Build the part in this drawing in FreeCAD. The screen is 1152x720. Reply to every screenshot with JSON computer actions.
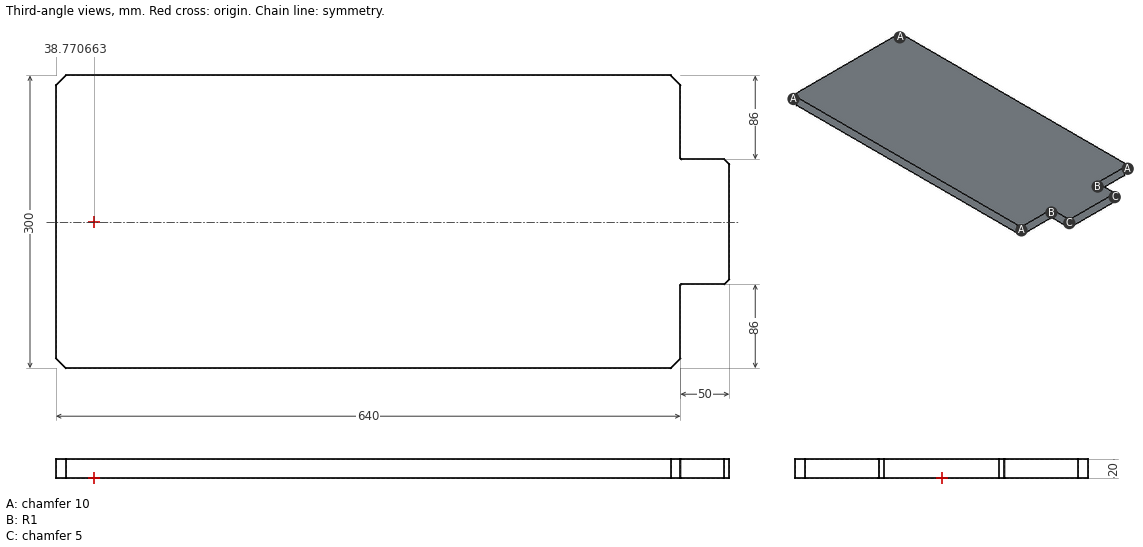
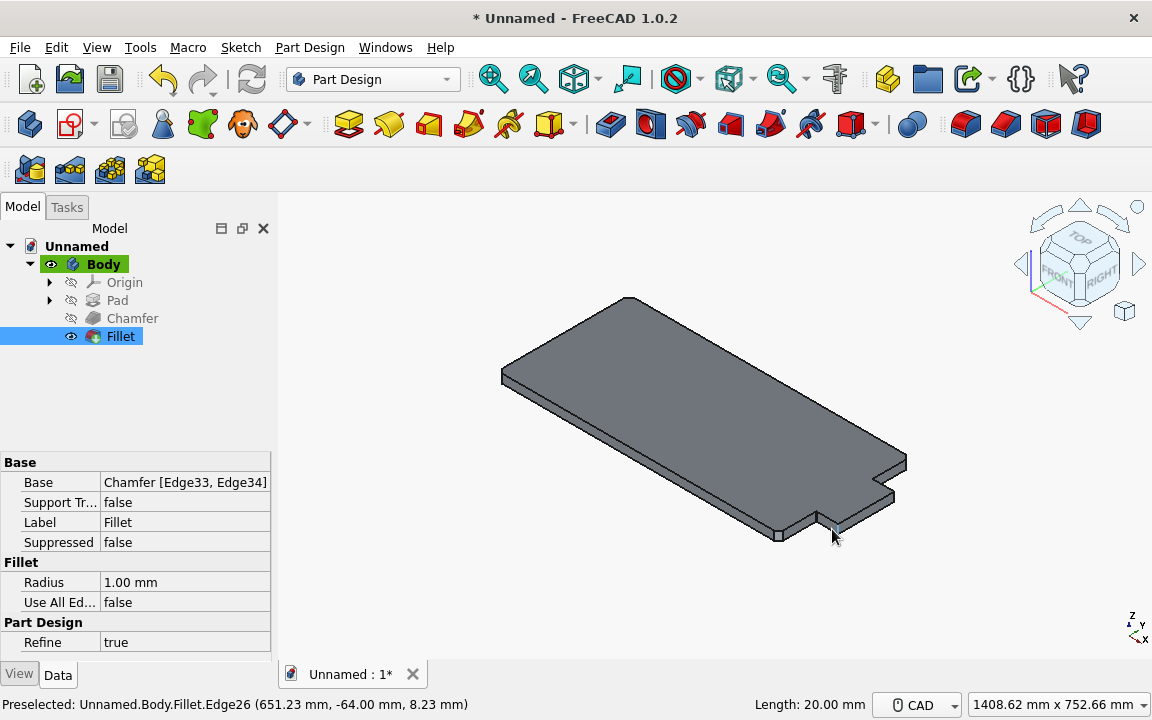
{"action": "scroll", "coordinate": [894, 496], "scroll_direction": "up", "scroll_amount": 6}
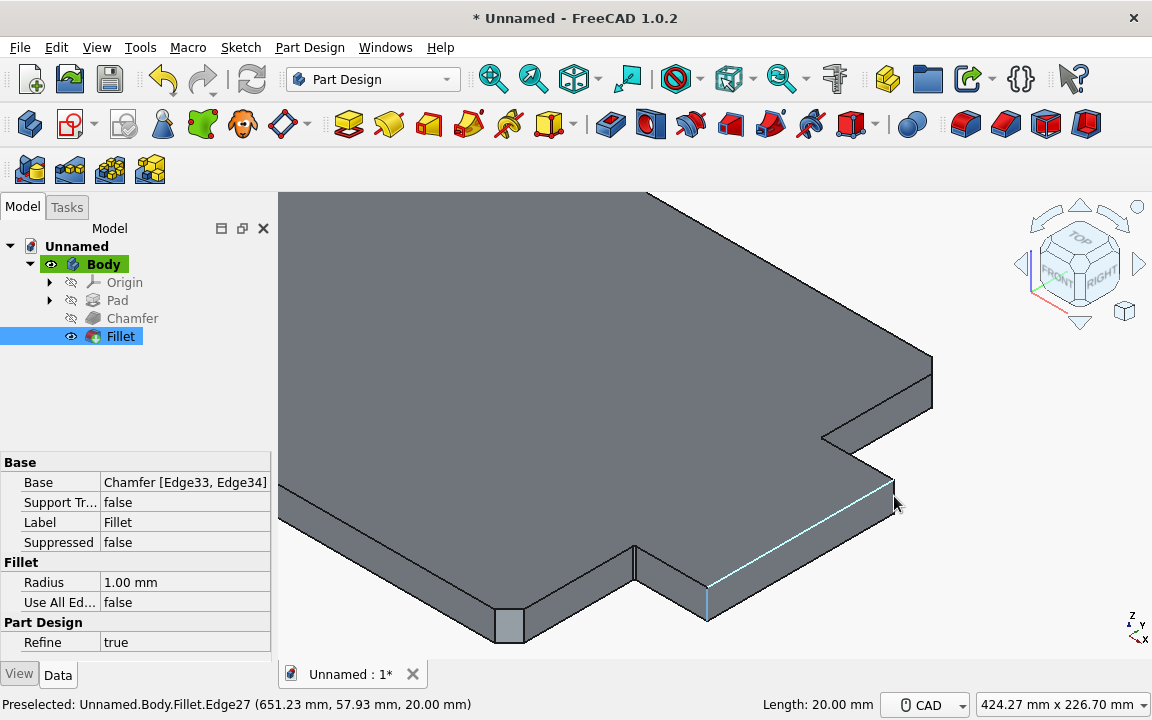
{"action": "left_click", "coordinate": [494, 80]}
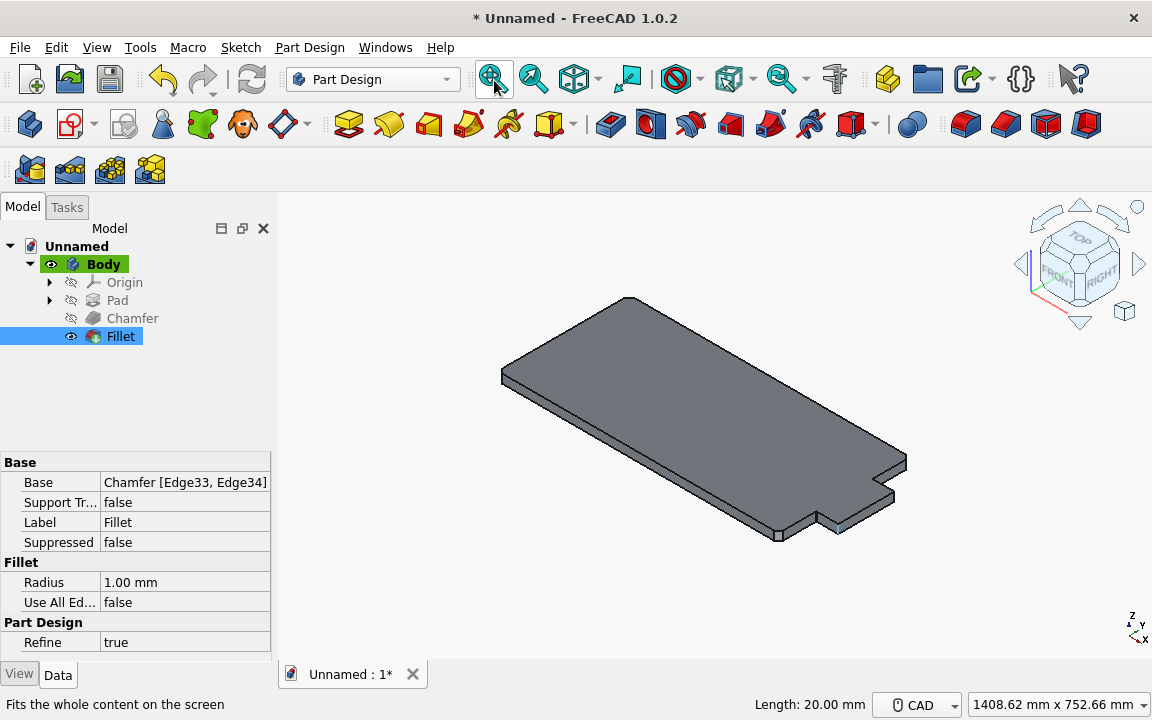
{"action": "key", "text": "2"}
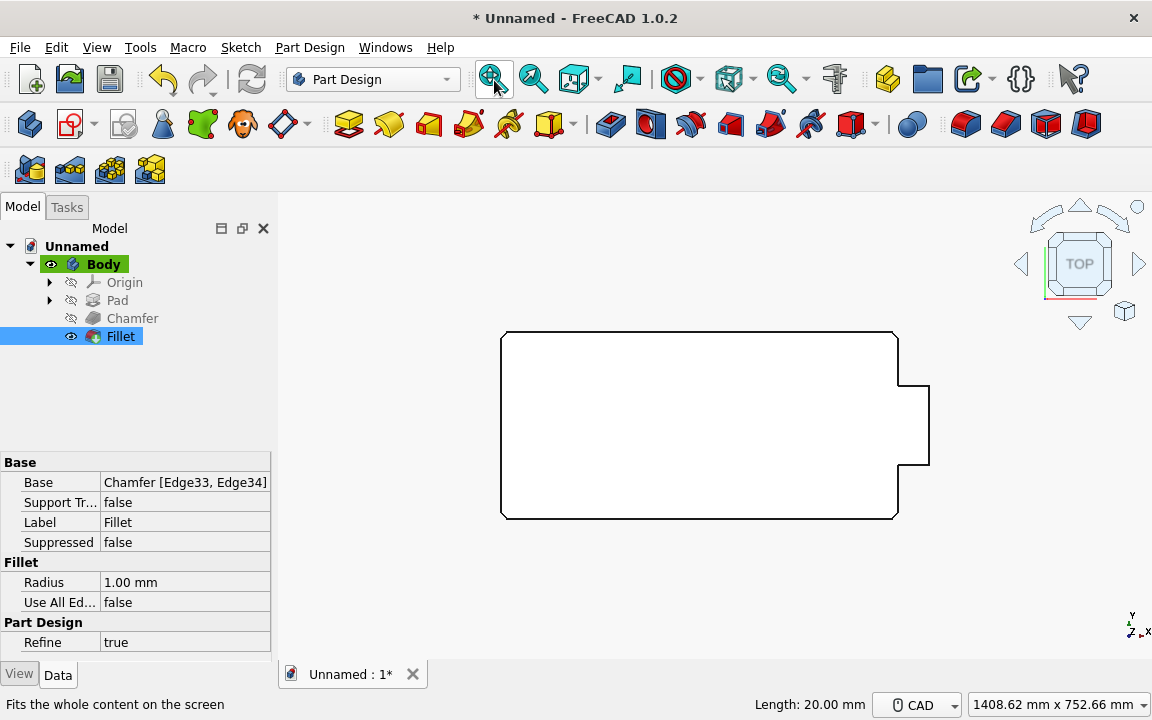
{"action": "scroll", "coordinate": [929, 385], "scroll_direction": "up", "scroll_amount": 6}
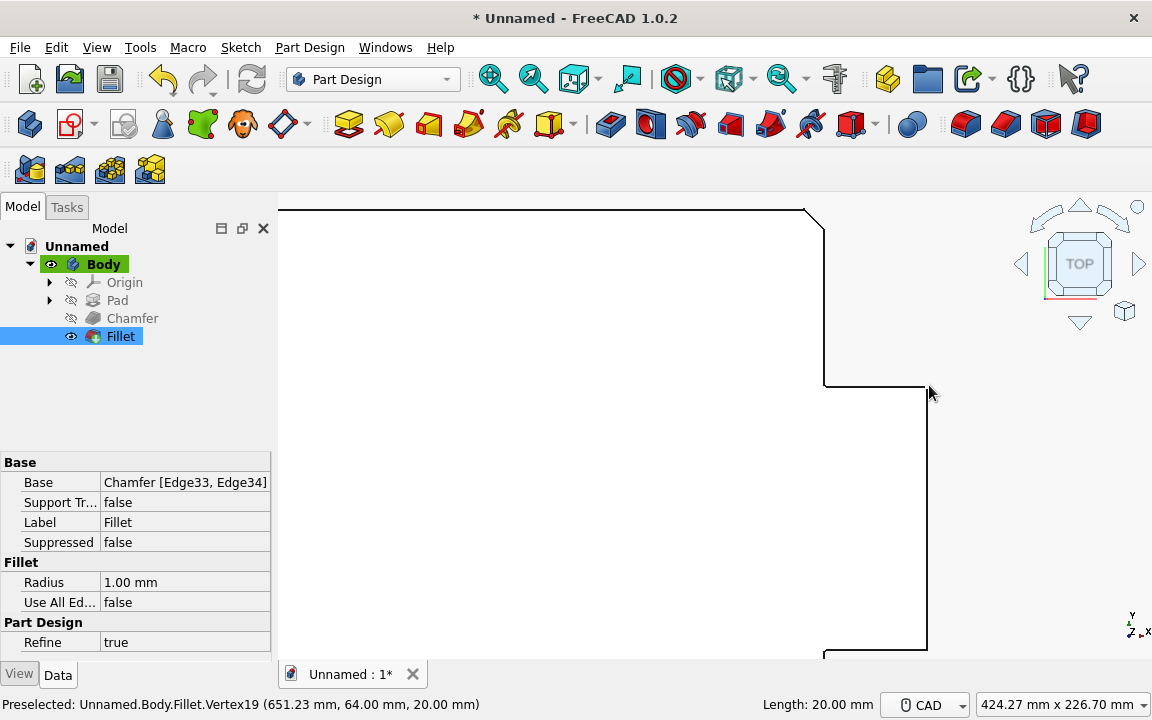
{"action": "left_click", "coordinate": [494, 80]}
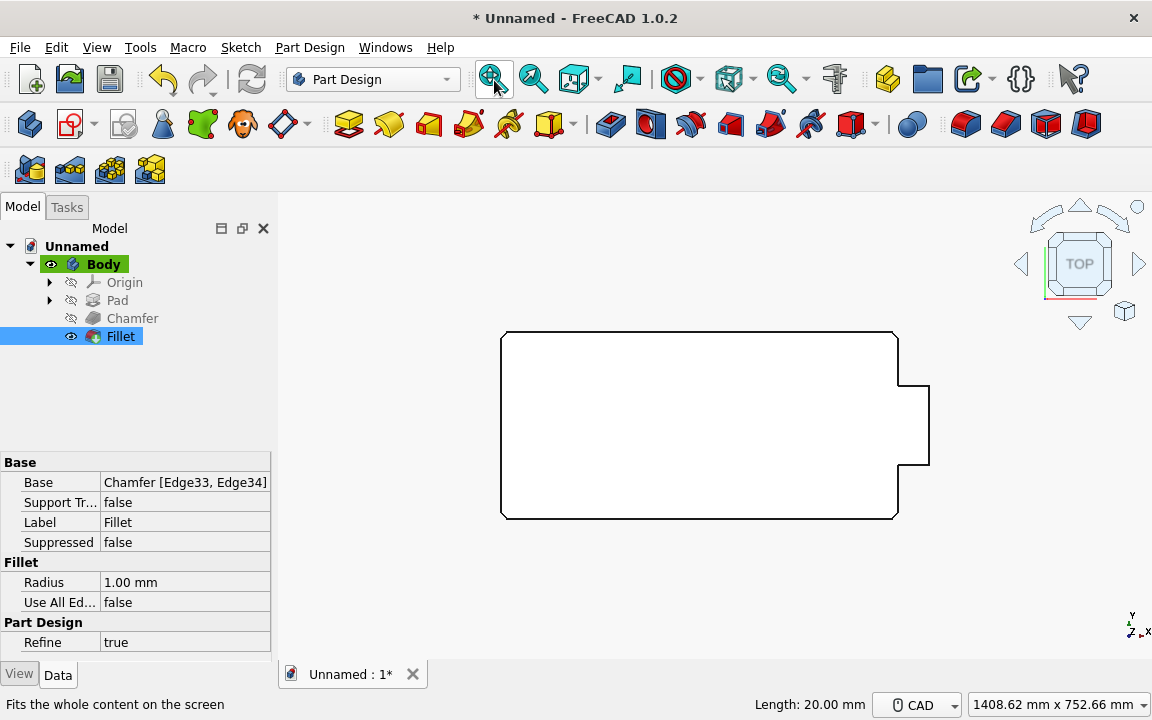
{"action": "key", "text": "0"}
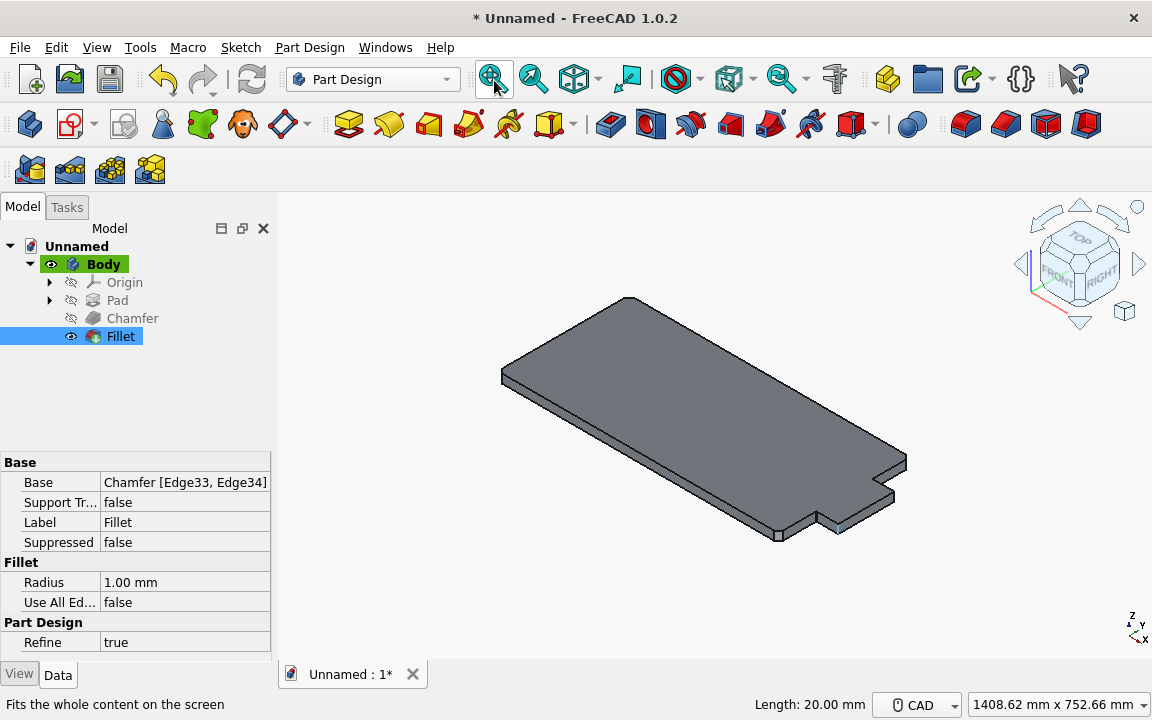
{"action": "scroll", "coordinate": [894, 496], "scroll_direction": "up", "scroll_amount": 6}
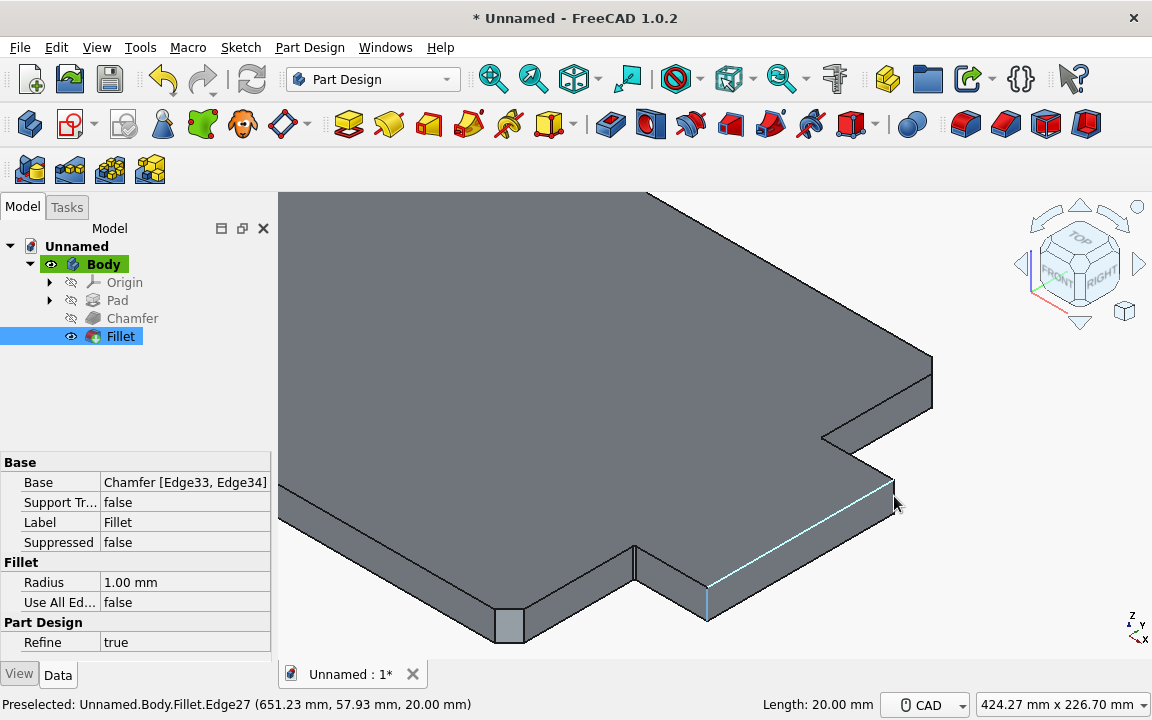
{"action": "left_click", "coordinate": [494, 80]}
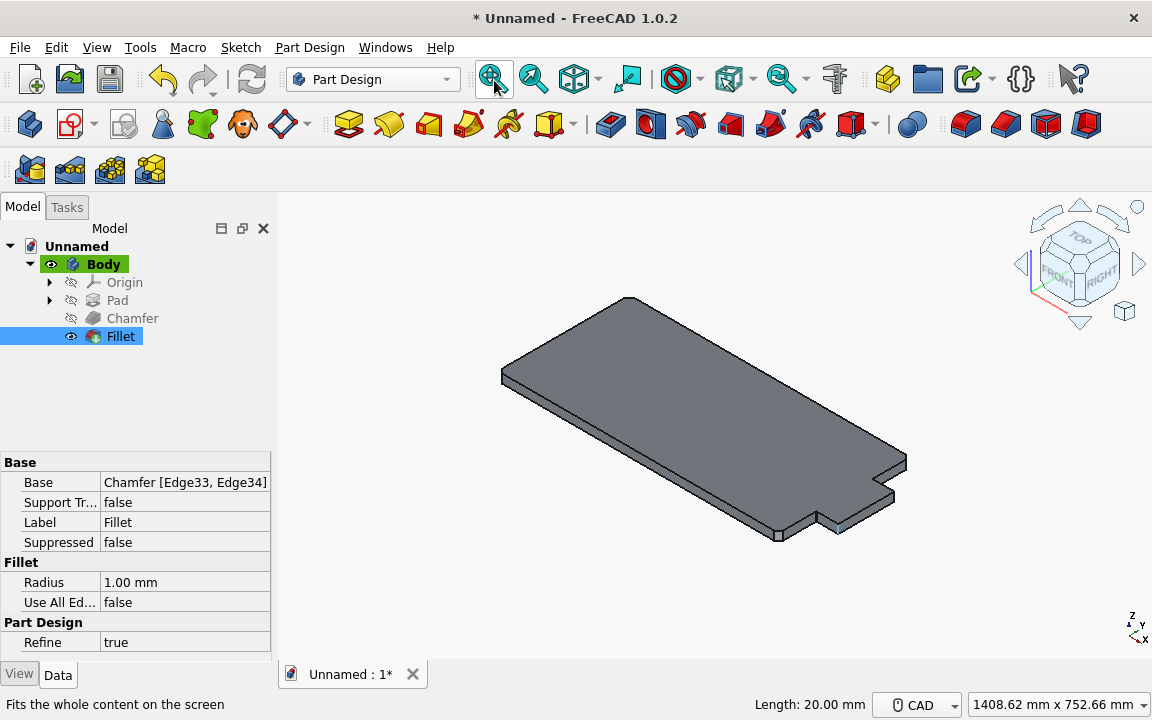
{"action": "key", "text": "1"}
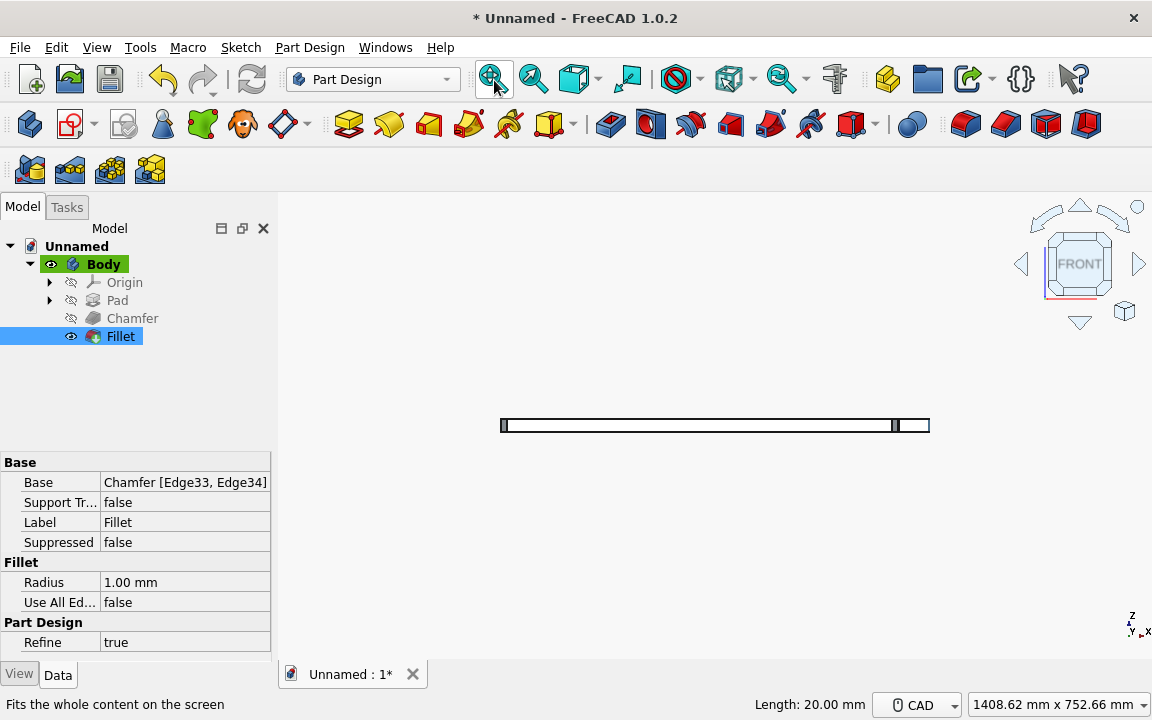
{"action": "scroll", "coordinate": [929, 424], "scroll_direction": "up", "scroll_amount": 6}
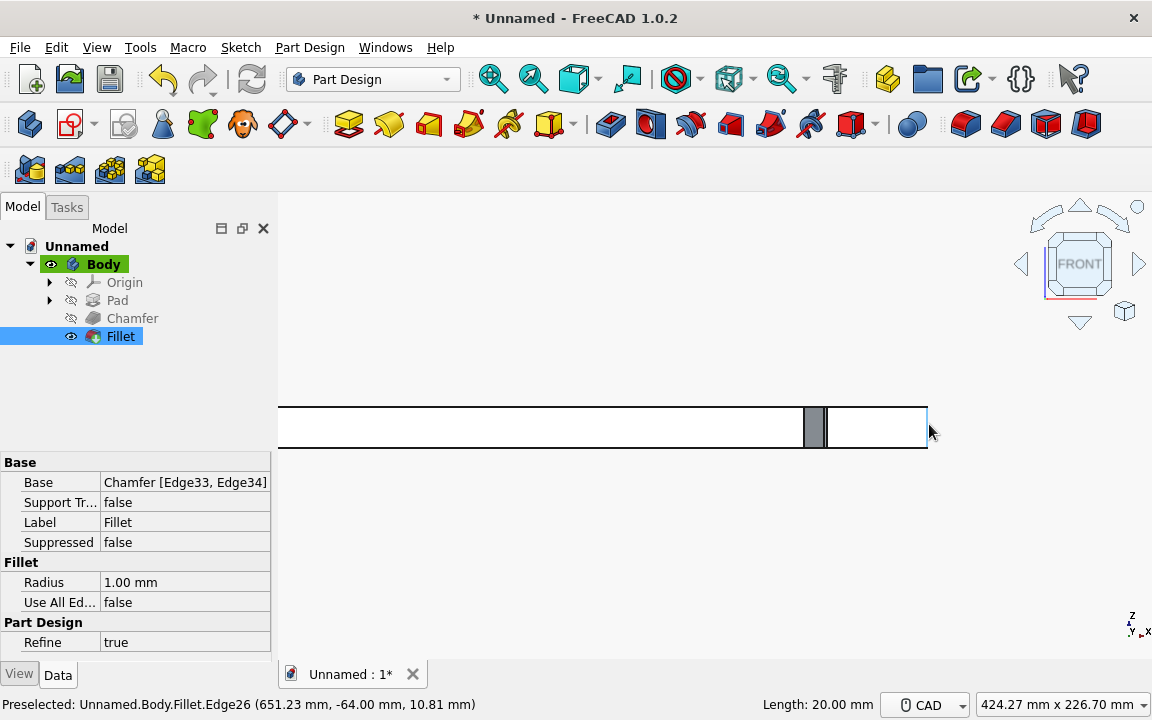
{"action": "left_click", "coordinate": [494, 80]}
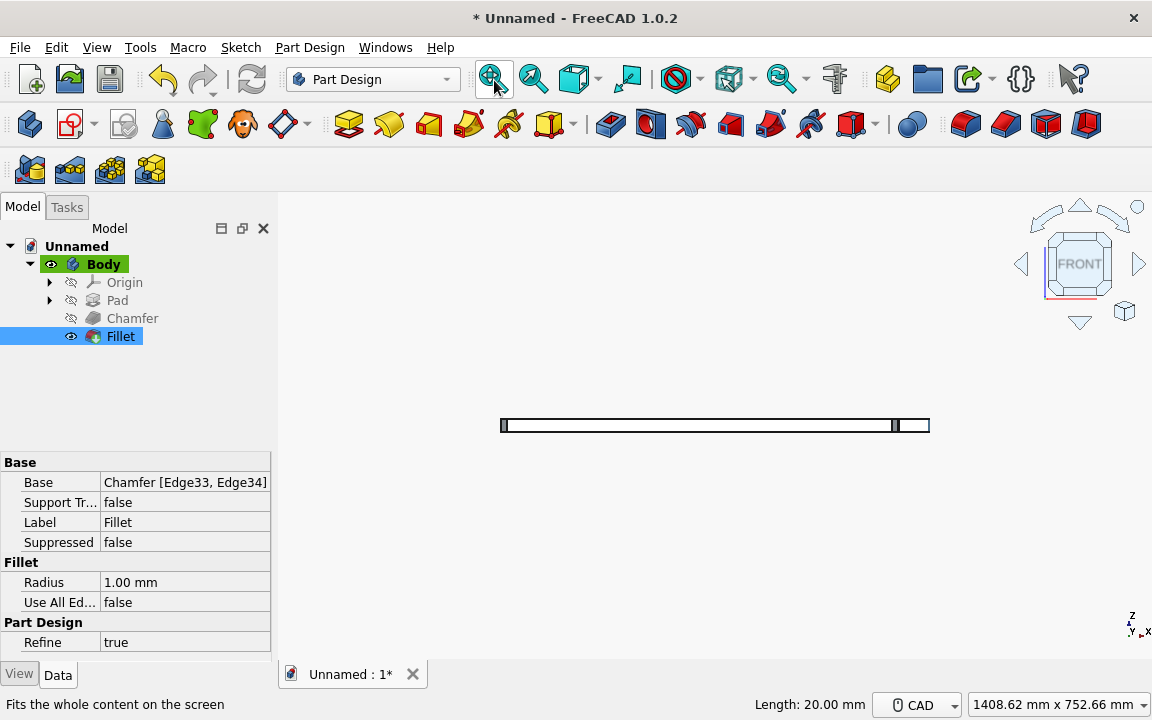
{"action": "key", "text": "3"}